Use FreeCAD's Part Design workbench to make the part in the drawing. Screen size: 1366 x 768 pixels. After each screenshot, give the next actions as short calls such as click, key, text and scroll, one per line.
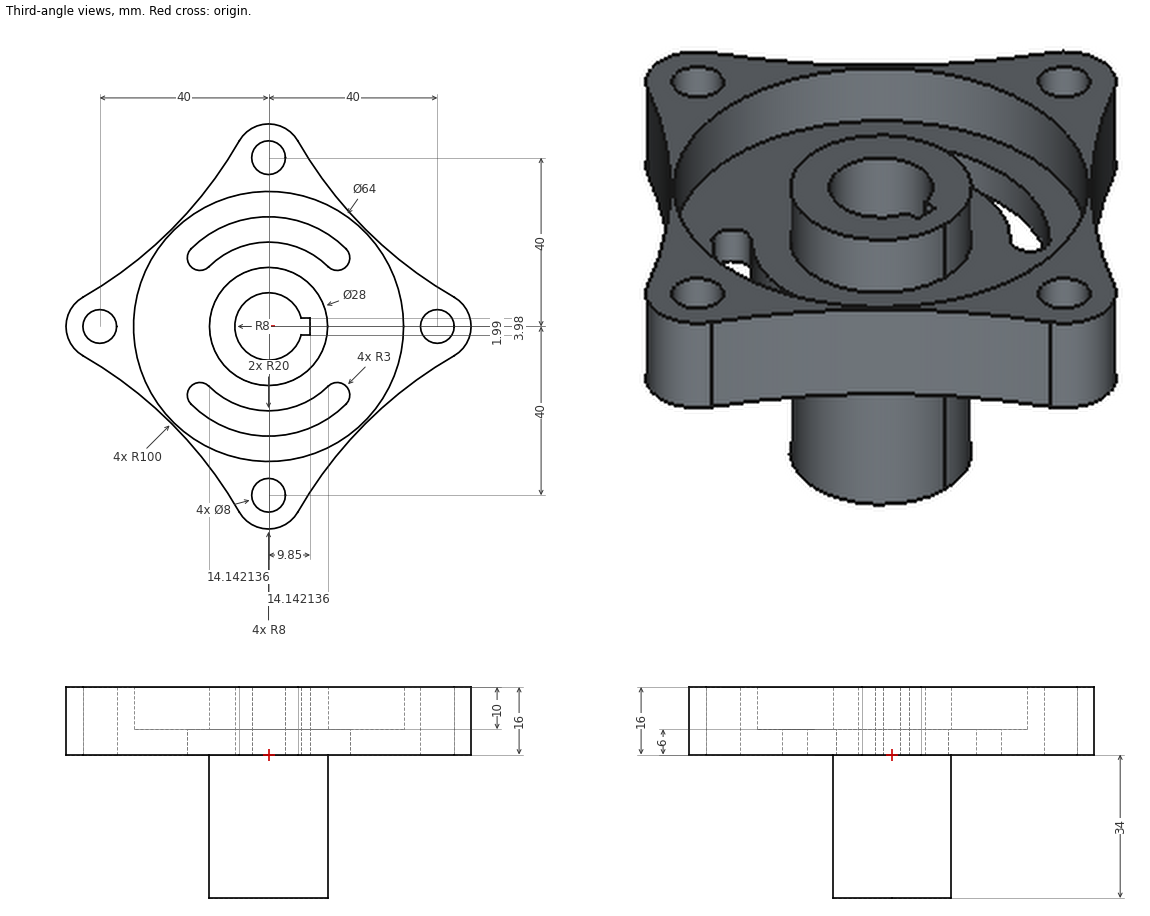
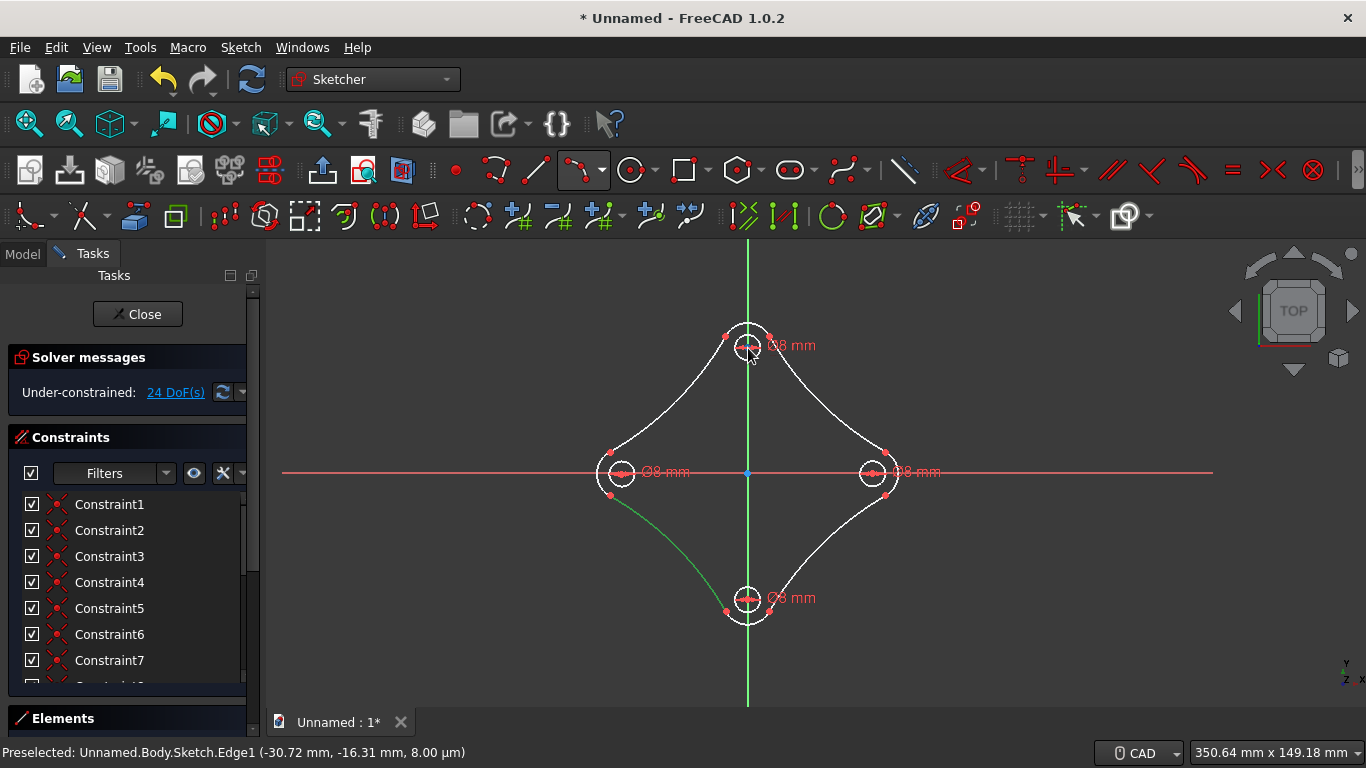
scroll(738, 622, up, 2)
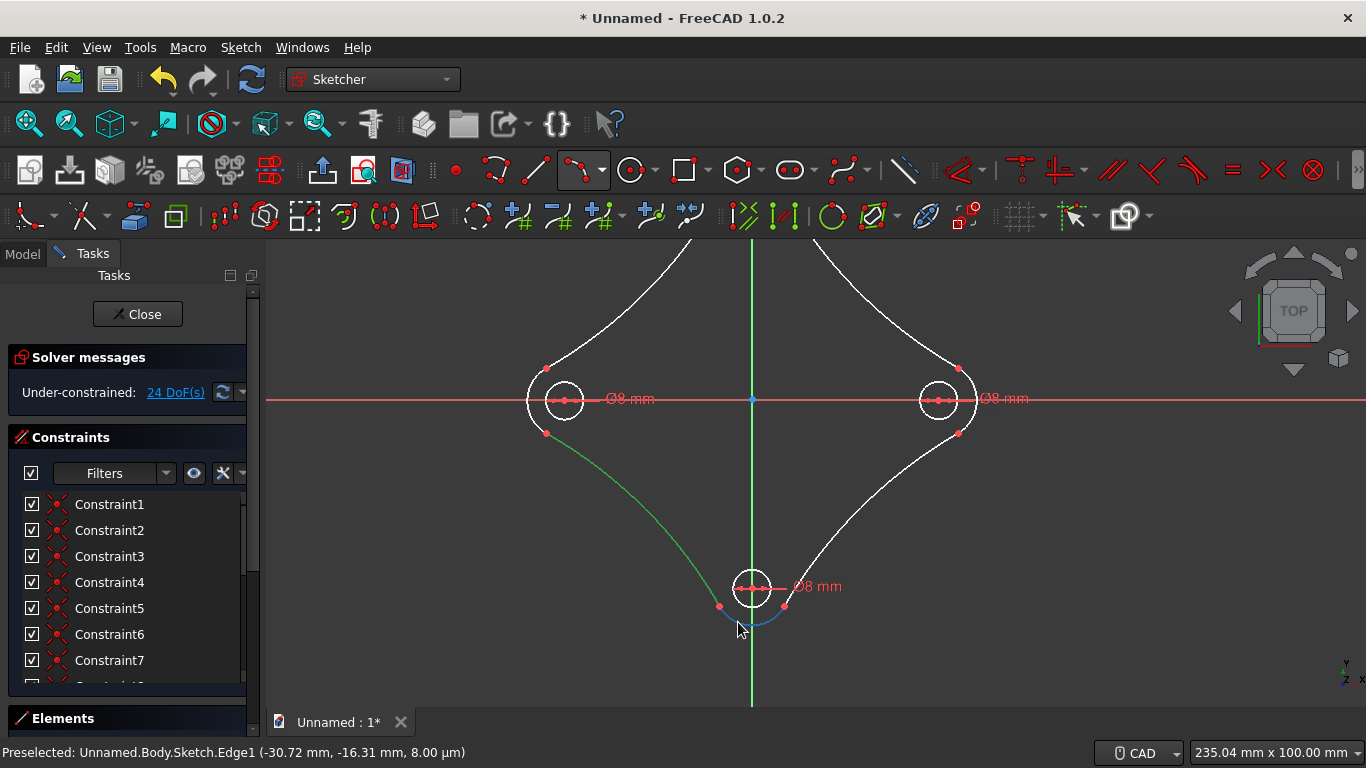
click(737, 622)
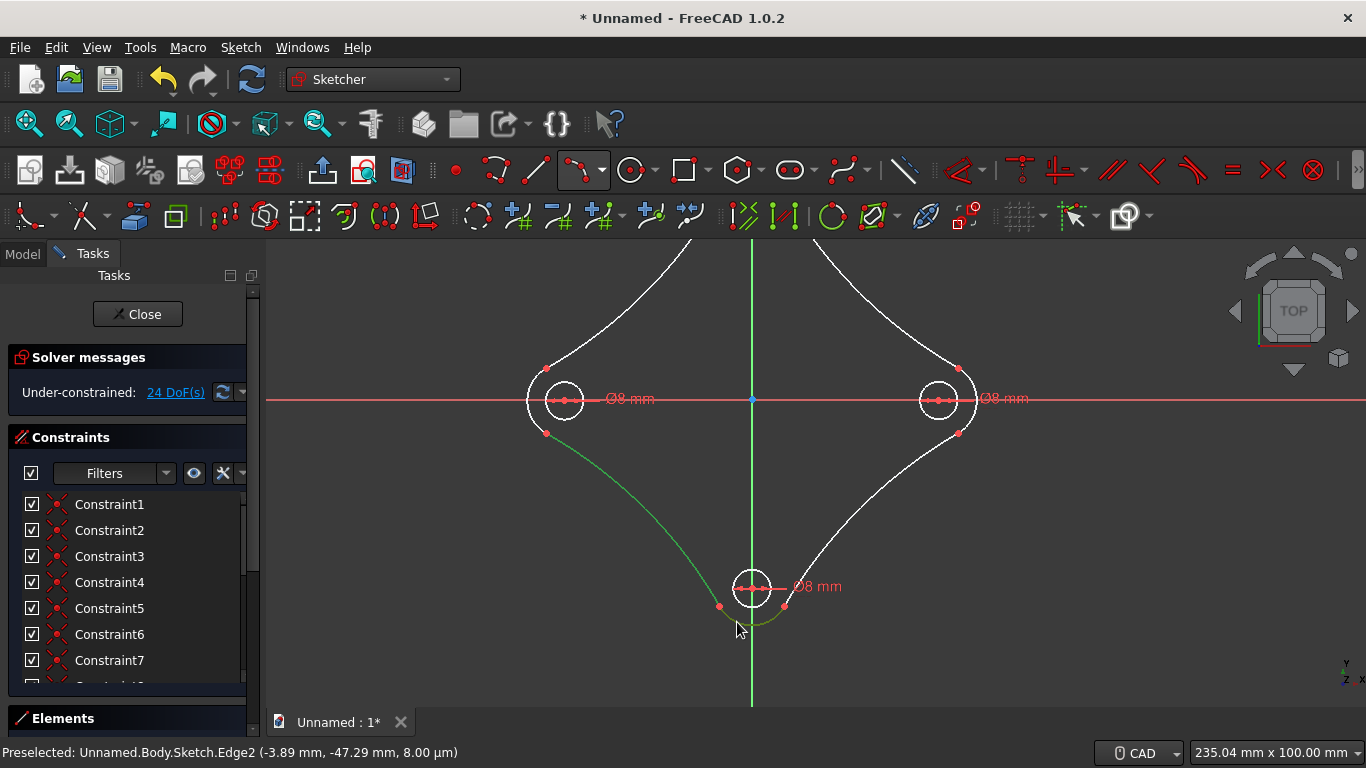
click(1194, 170)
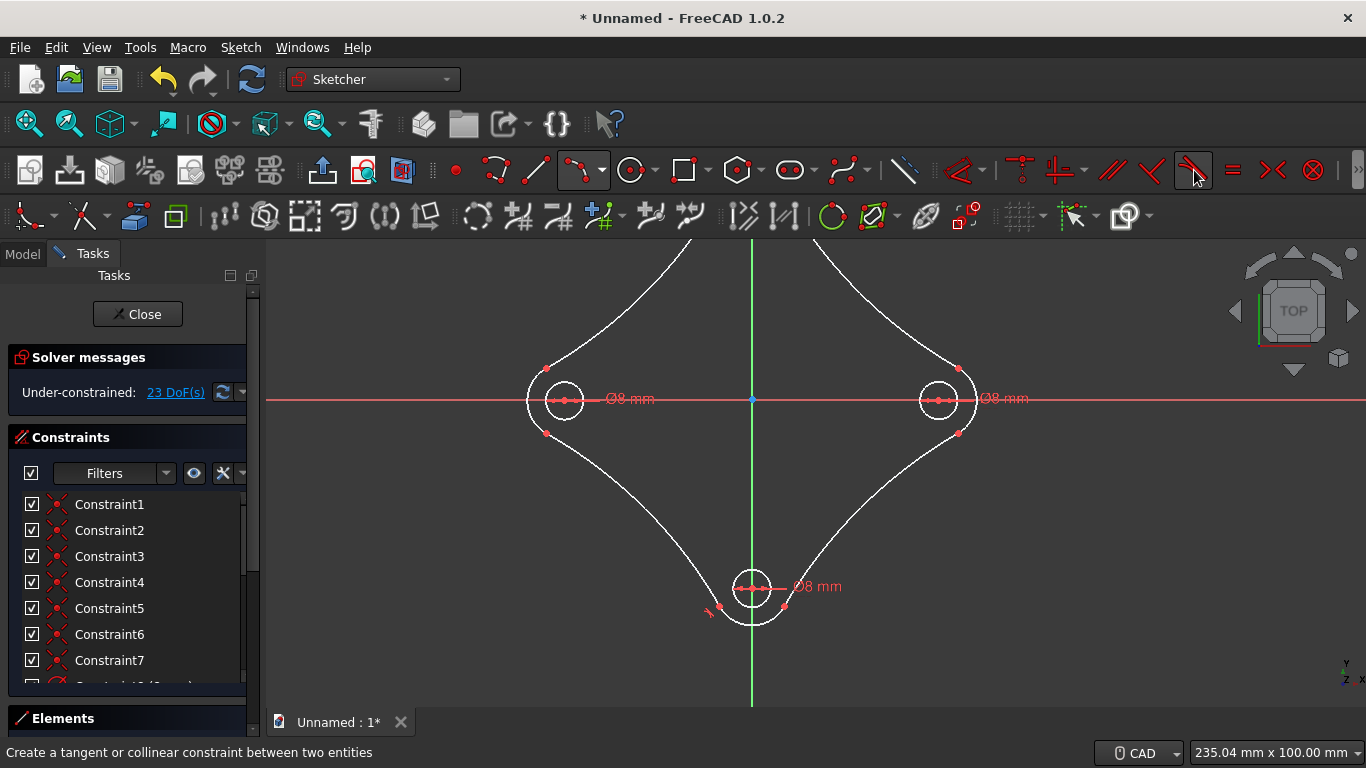
click(678, 545)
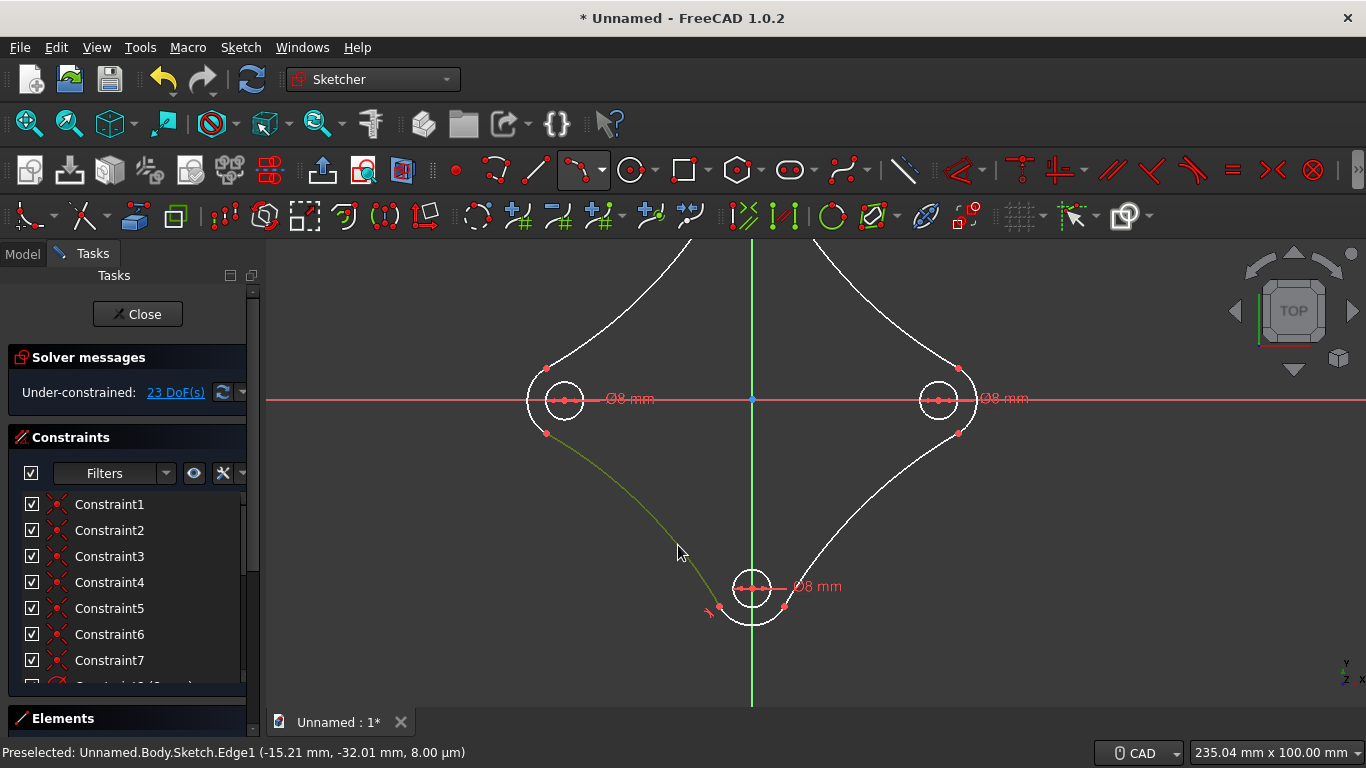
click(531, 385)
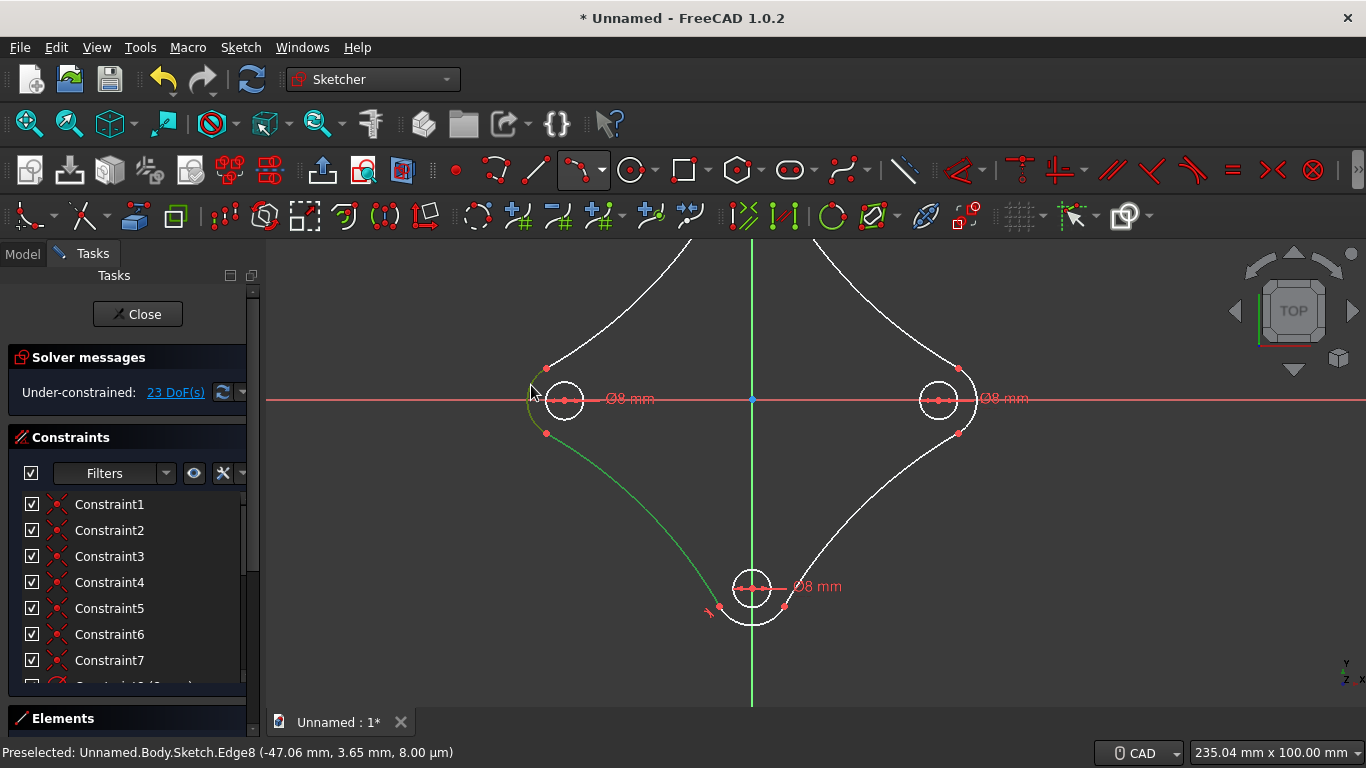
key(t)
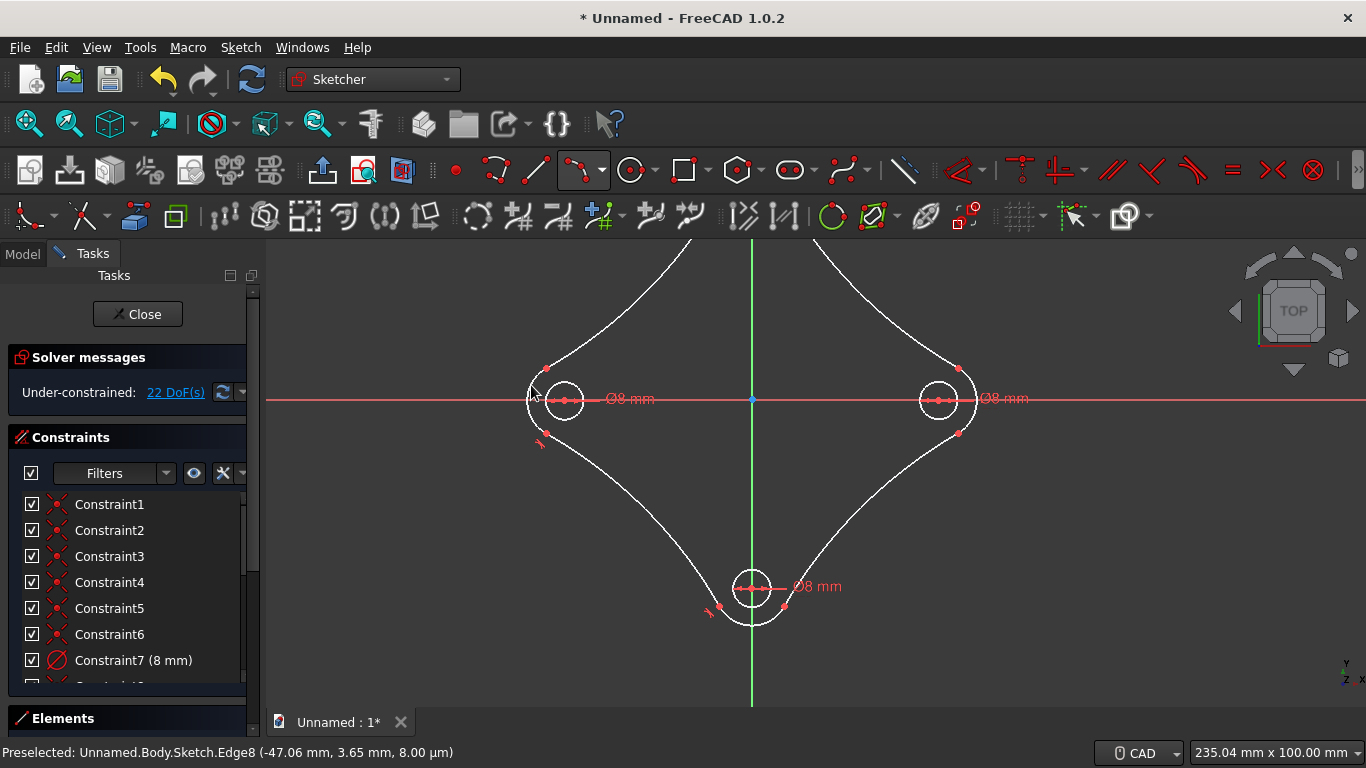
click(737, 622)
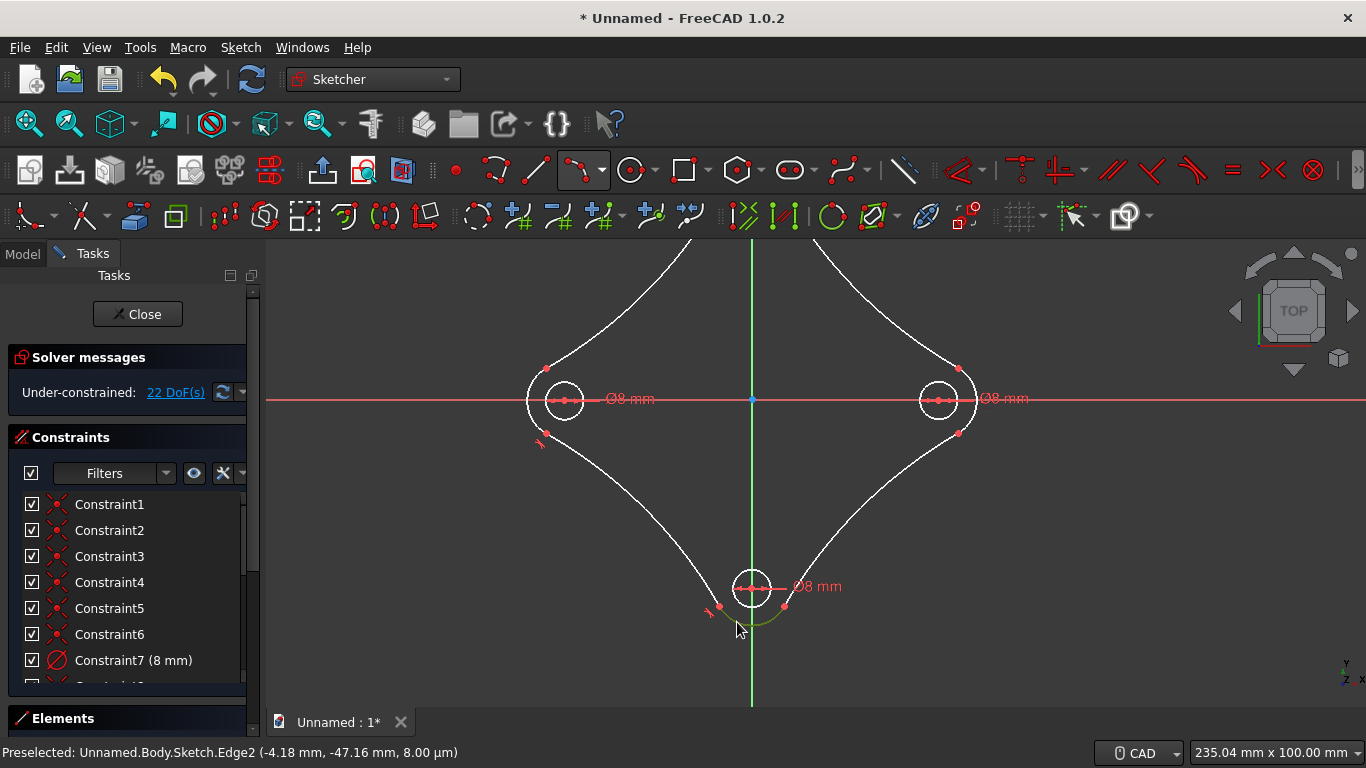
click(897, 475)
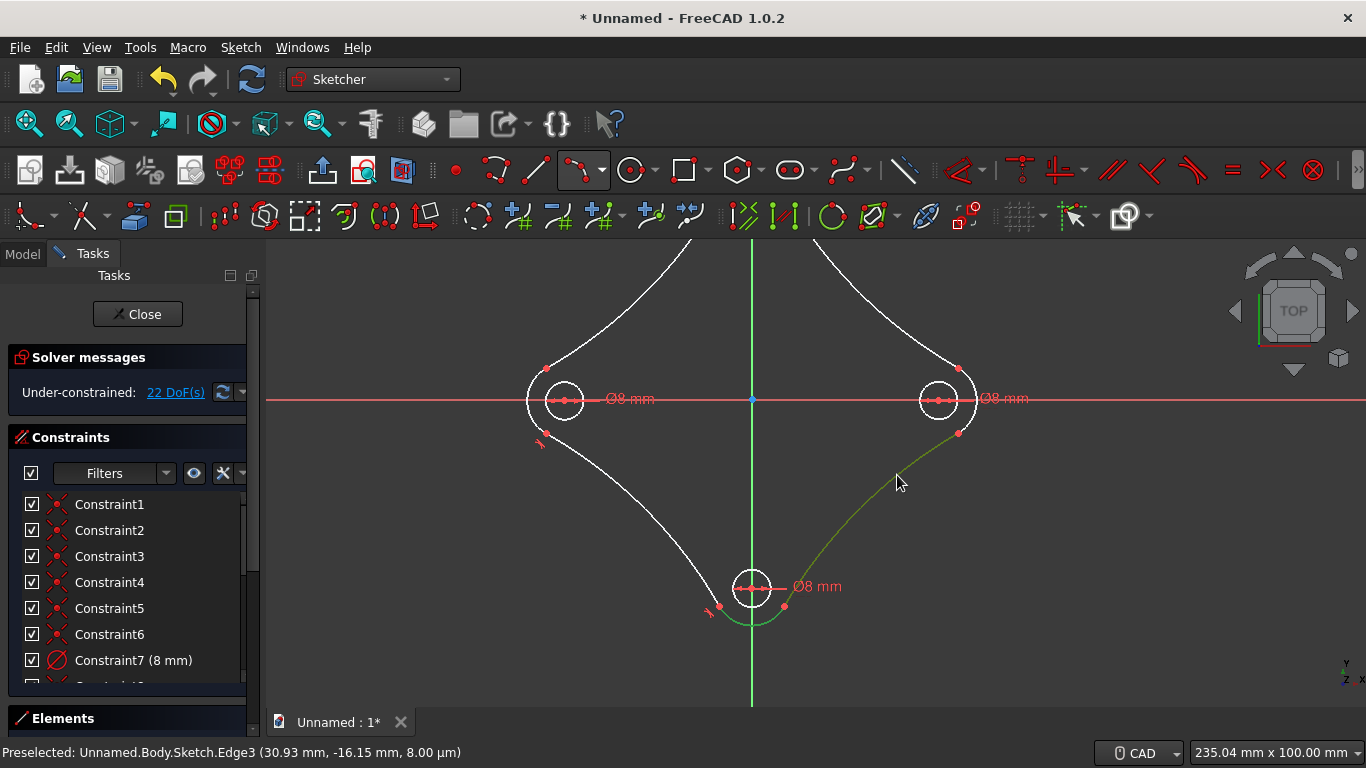
key(t)